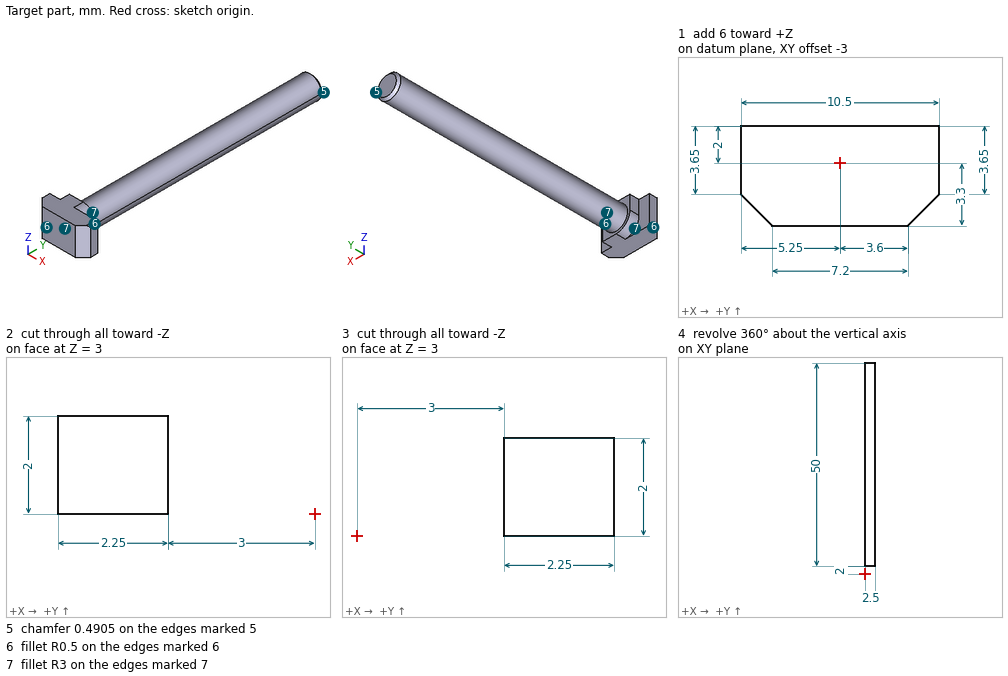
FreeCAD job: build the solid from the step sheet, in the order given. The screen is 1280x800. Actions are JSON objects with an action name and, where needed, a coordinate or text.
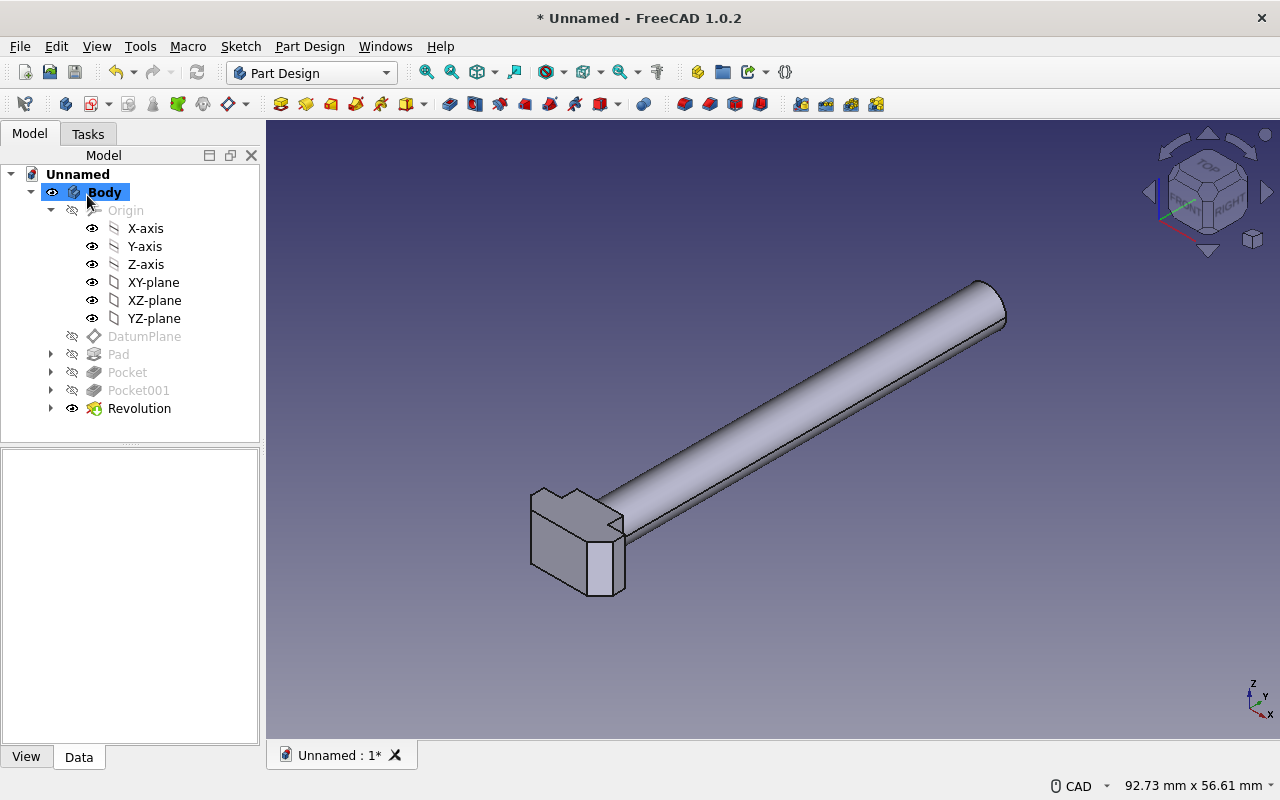
{"action": "key", "text": "2"}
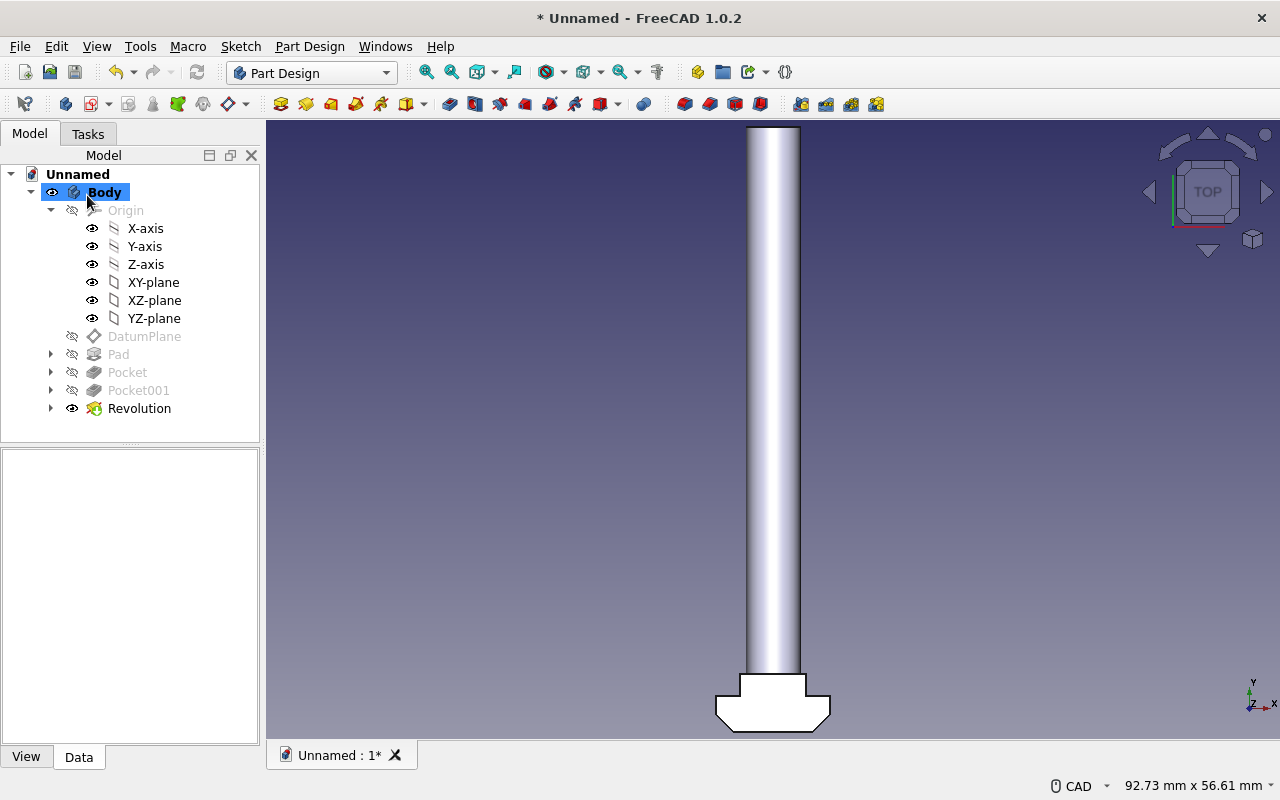
{"action": "key", "text": "1"}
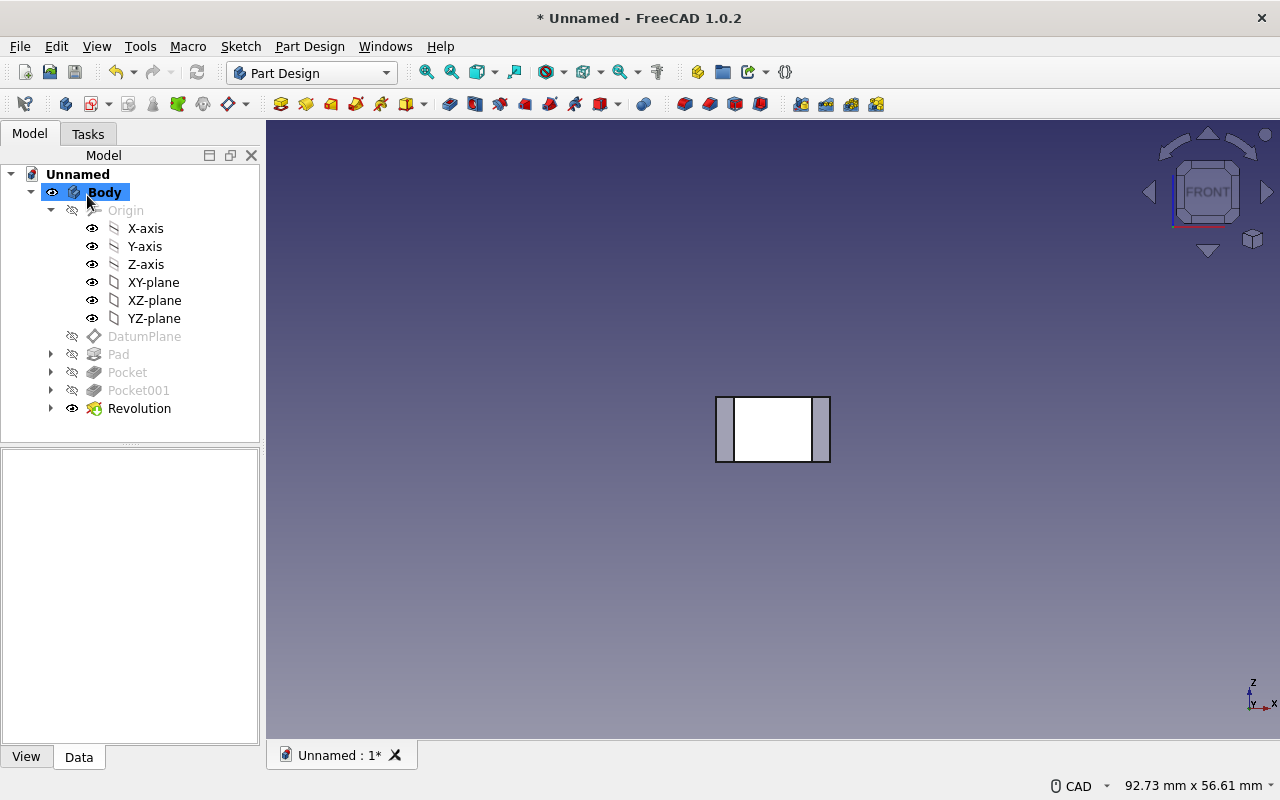
{"action": "key", "text": "v f"}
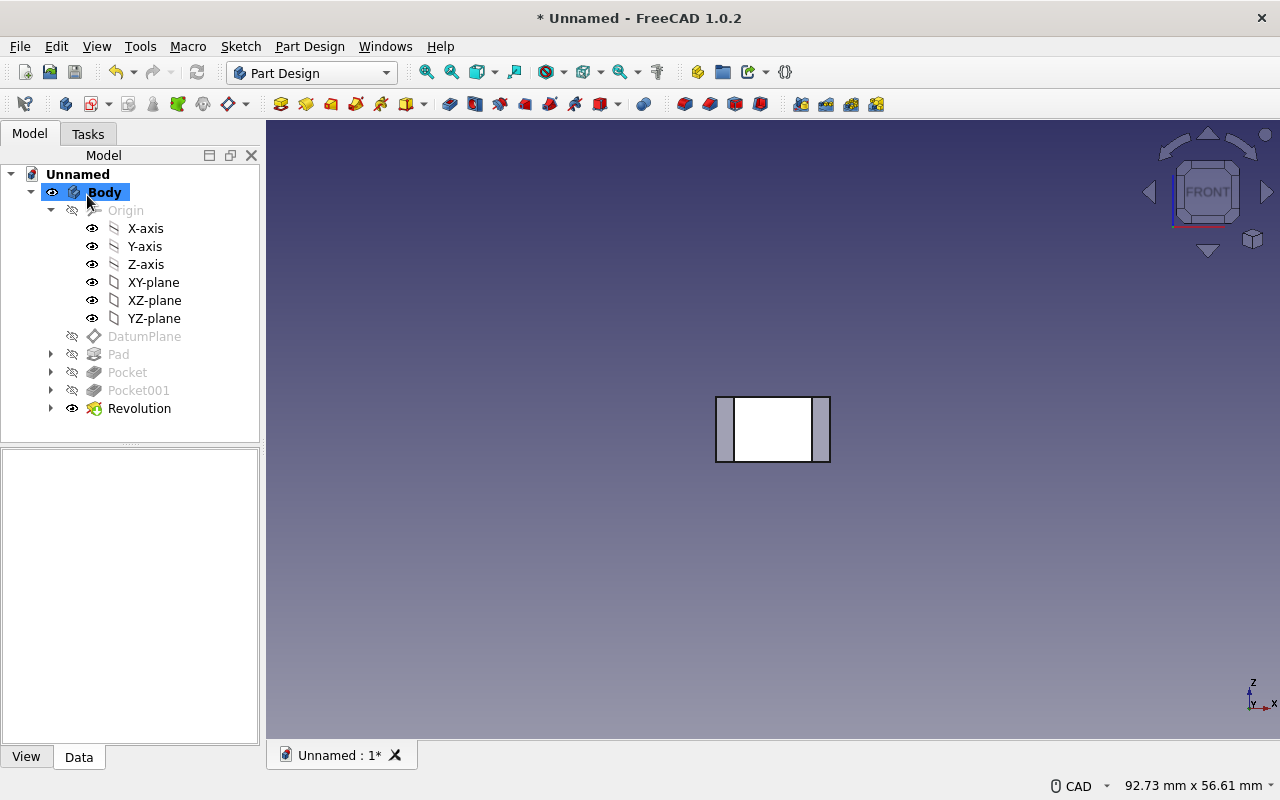
{"action": "key", "text": "3"}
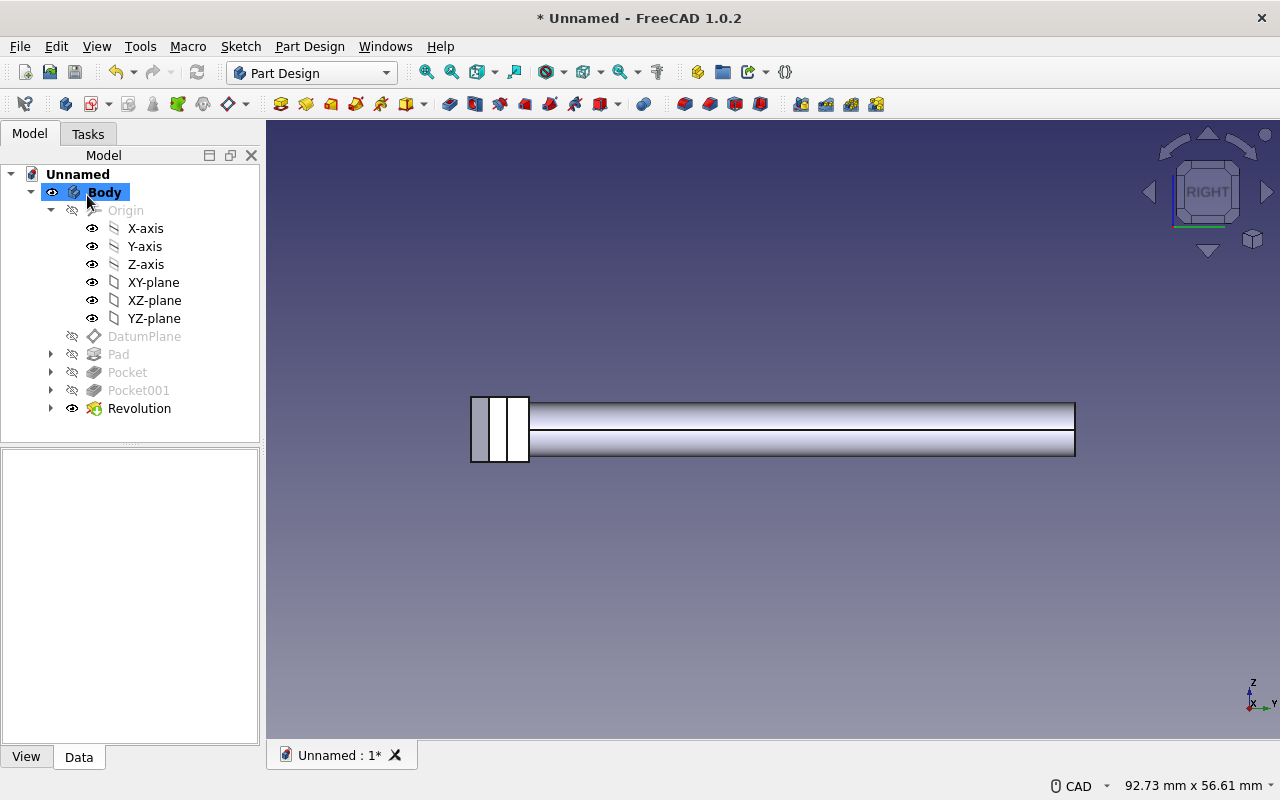
{"action": "left_click", "coordinate": [1075, 412]}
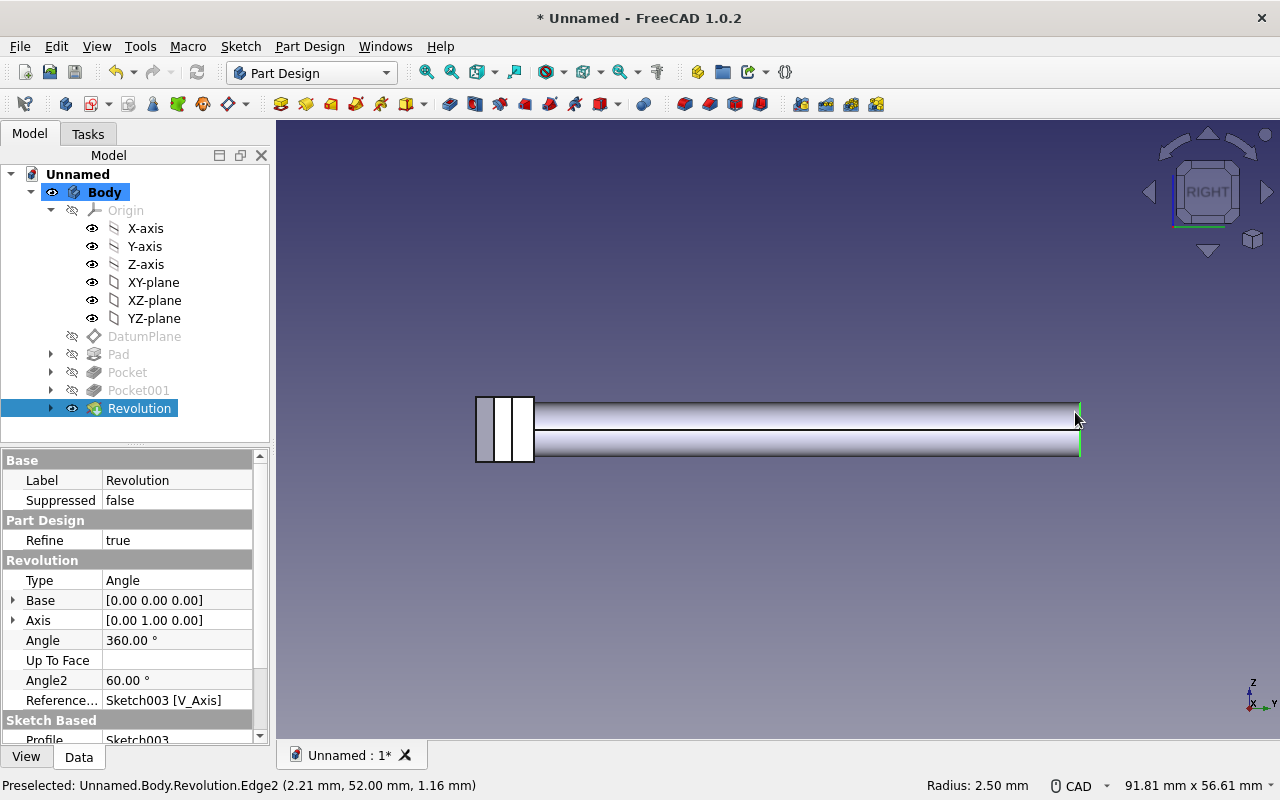
{"action": "left_click", "coordinate": [710, 104]}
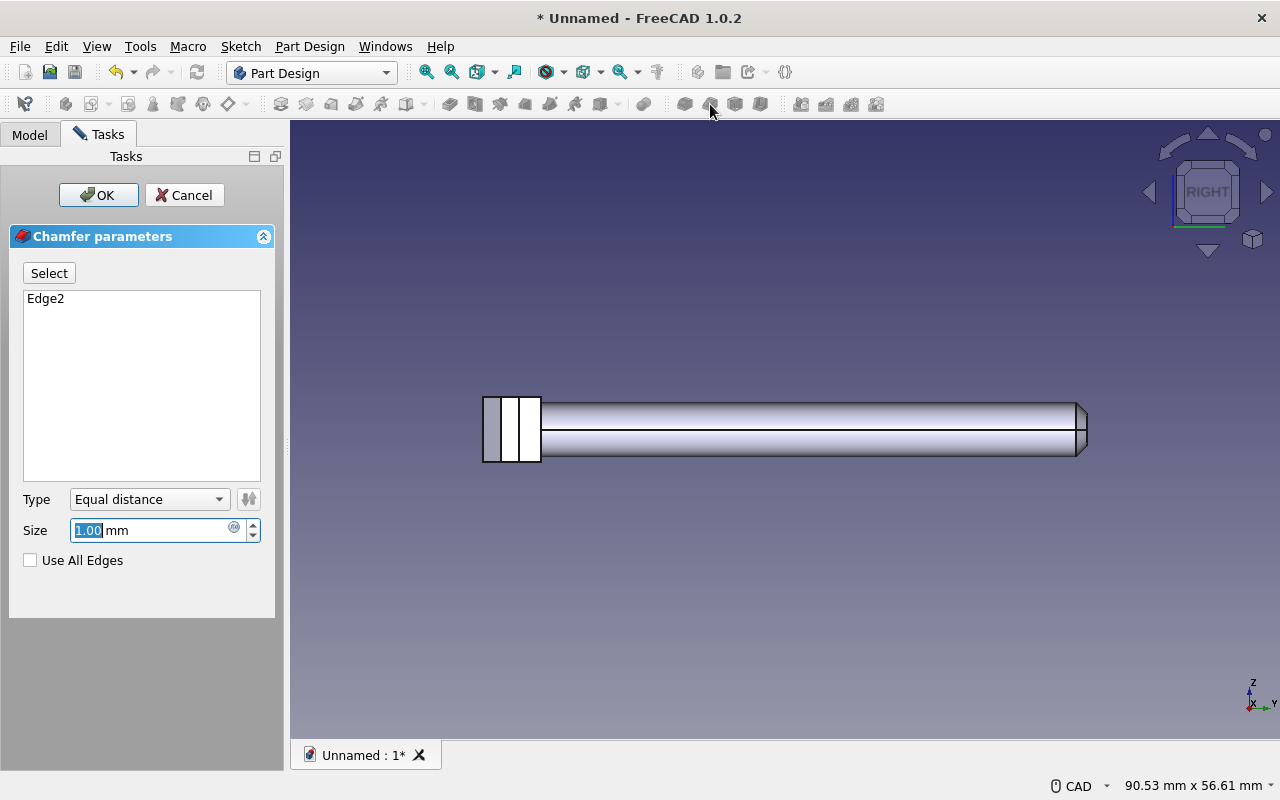
{"action": "type", "text": "0.4905"}
{"action": "key", "text": "Tab"}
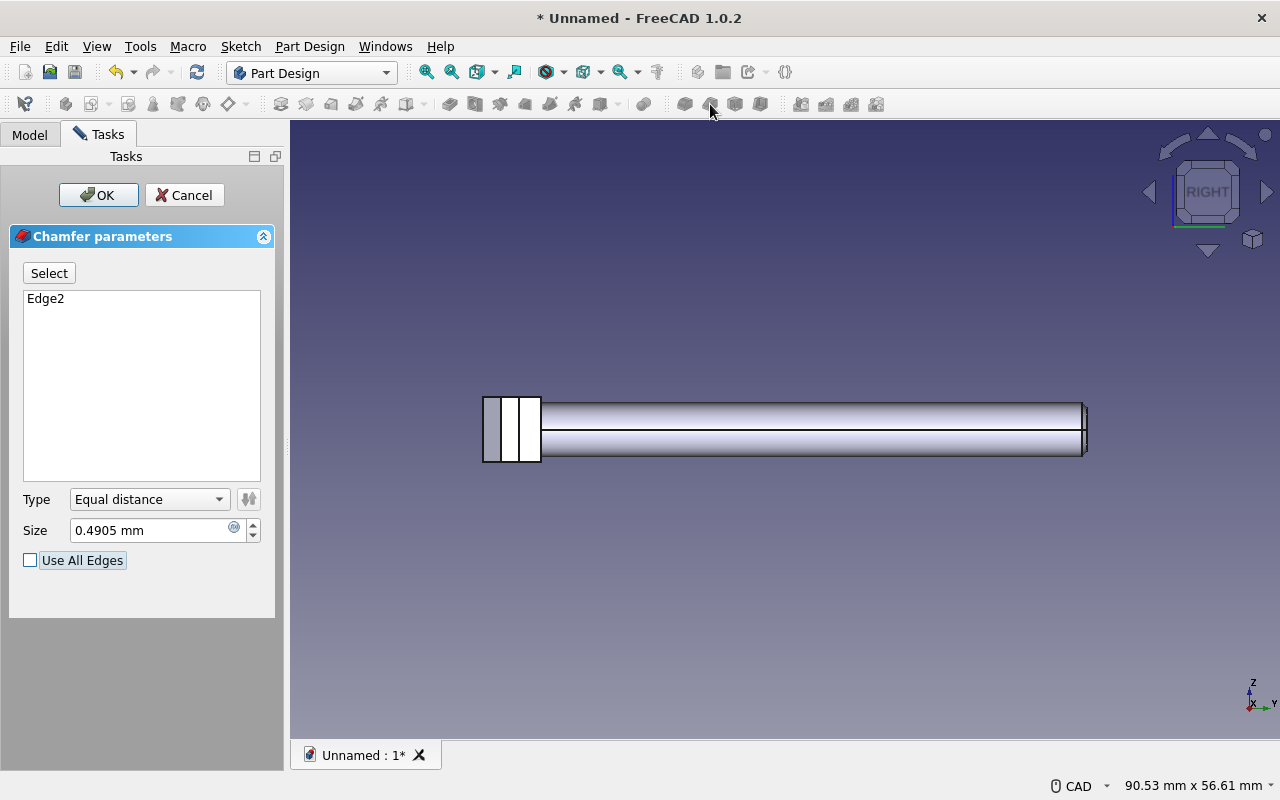
{"action": "left_click", "coordinate": [99, 195]}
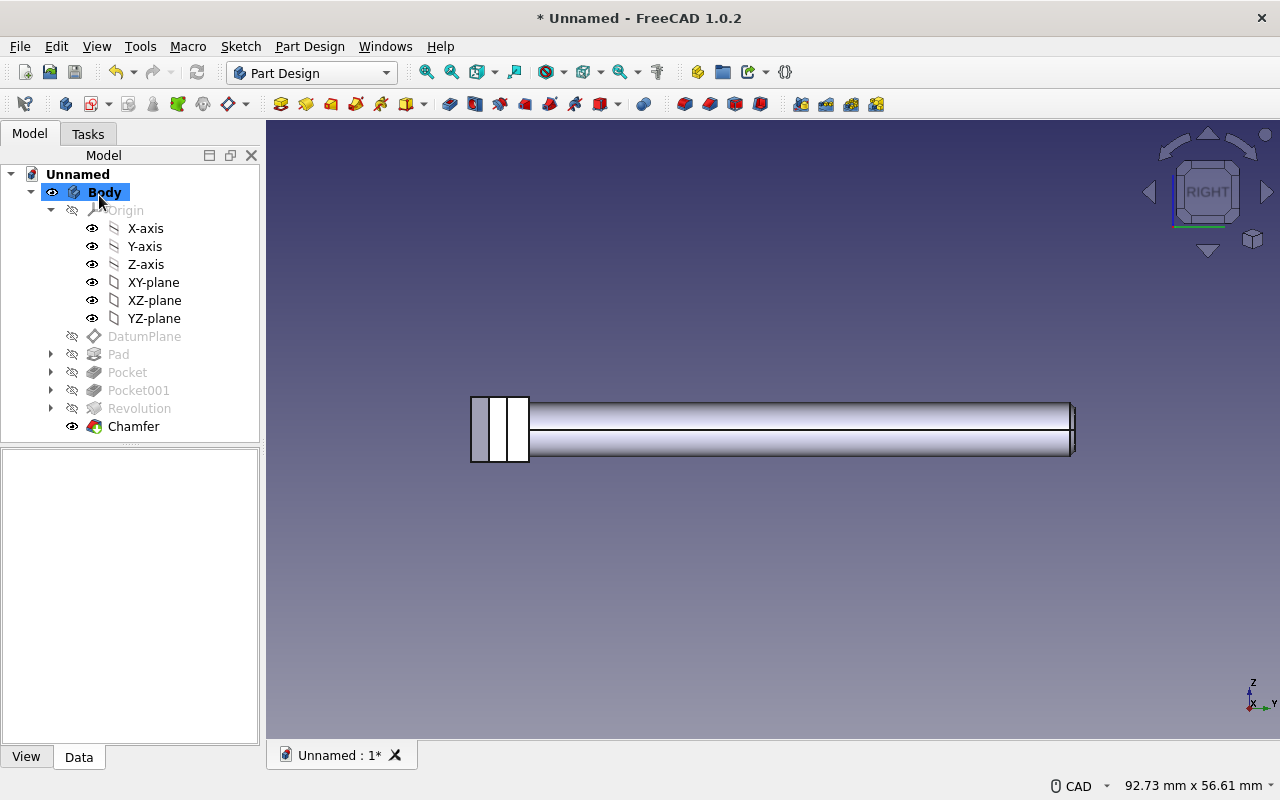
{"action": "left_click", "coordinate": [498, 396]}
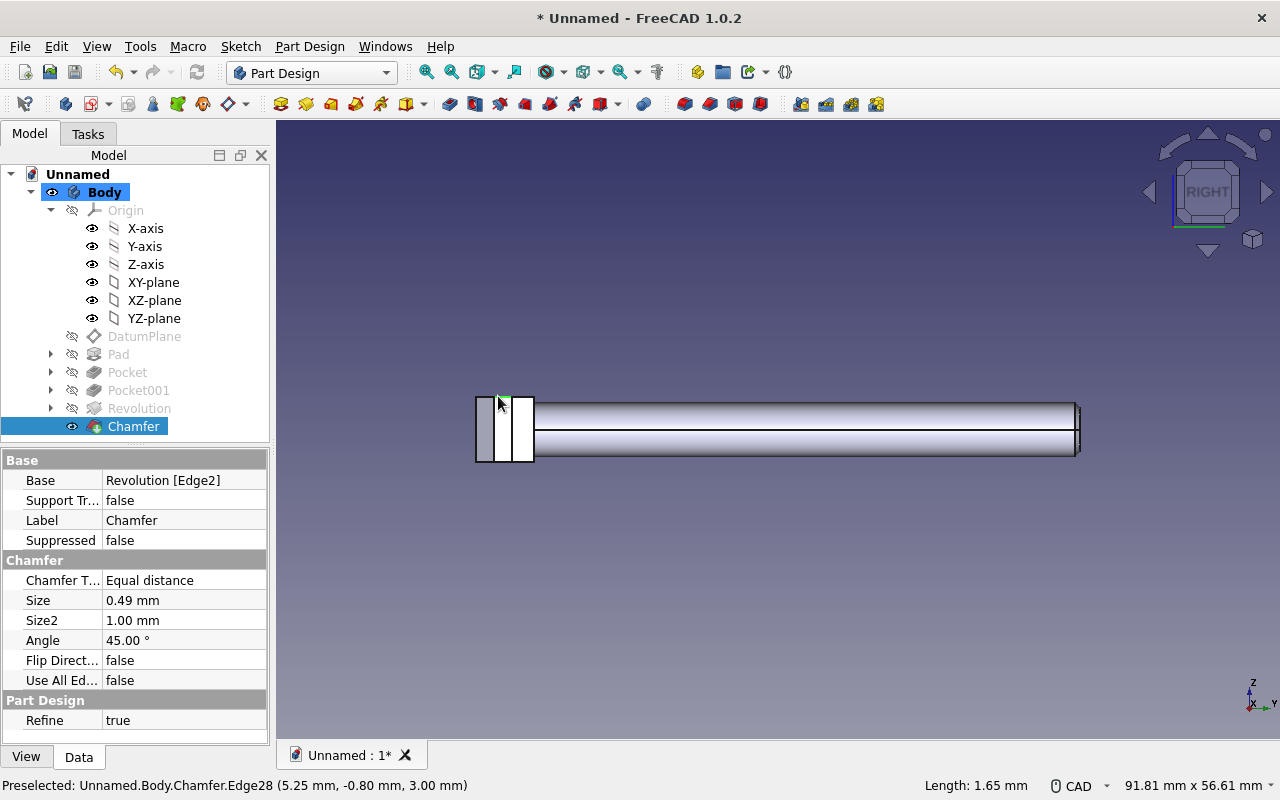
{"action": "scroll", "coordinate": [503, 461], "scroll_direction": "up", "scroll_amount": 4}